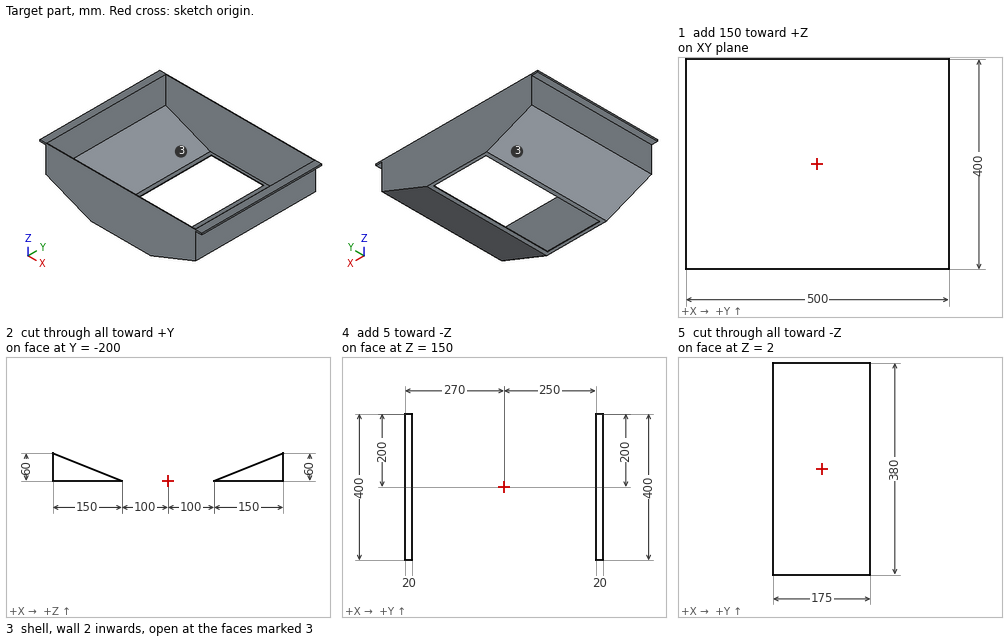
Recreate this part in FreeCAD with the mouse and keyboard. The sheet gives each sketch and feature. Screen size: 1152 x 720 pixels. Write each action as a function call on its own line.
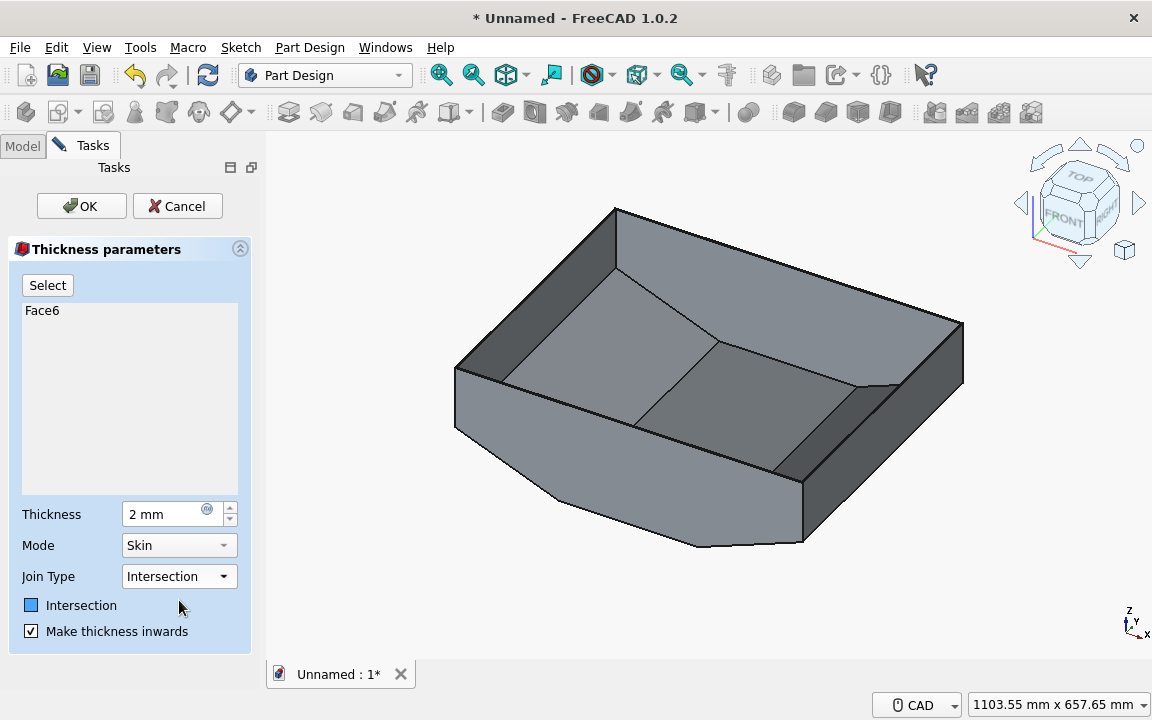
click(82, 206)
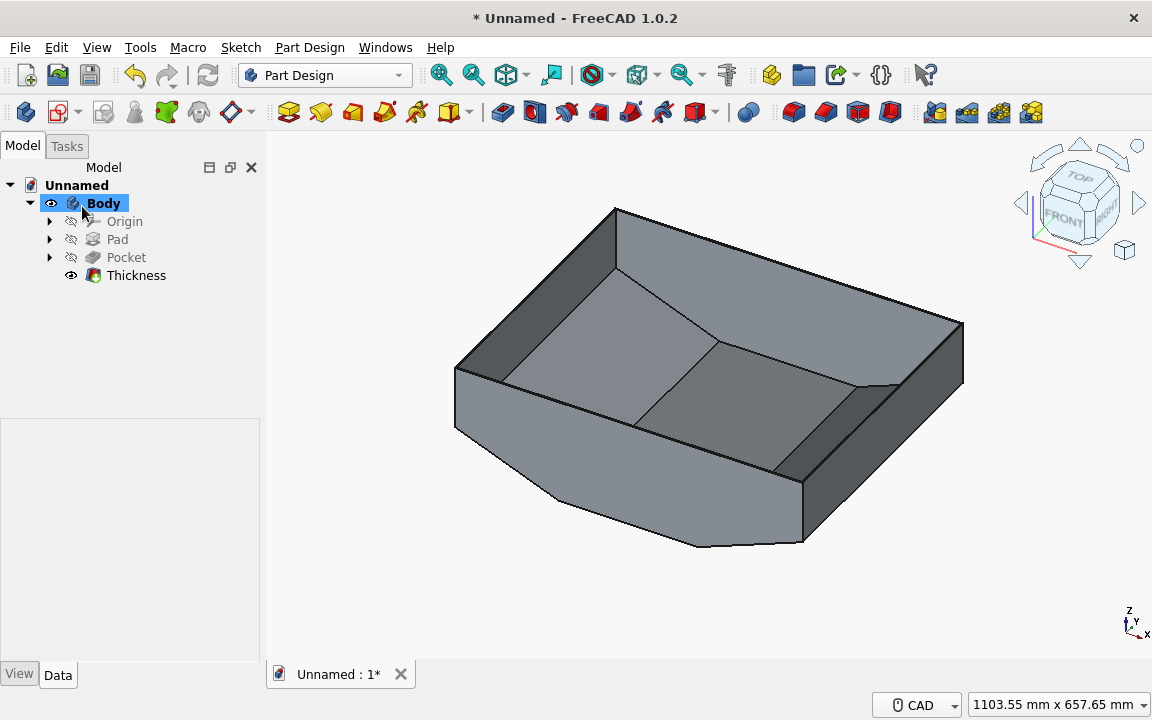
scroll(856, 428, up, 15)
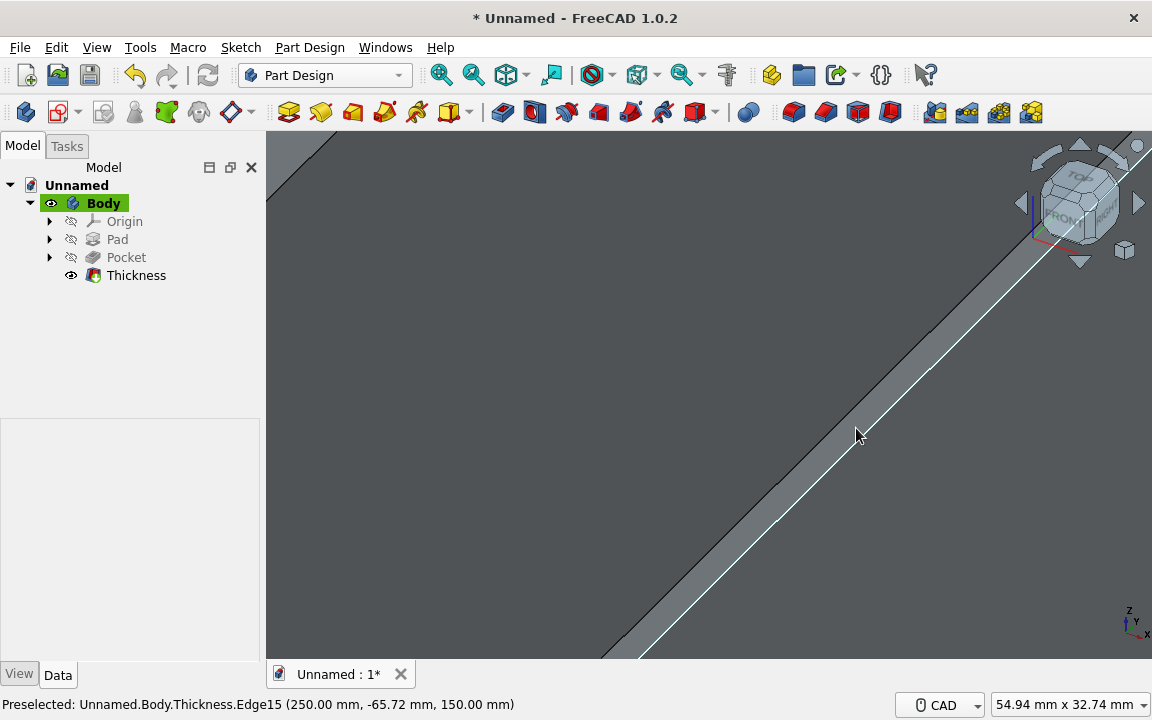
key(v)
key(f)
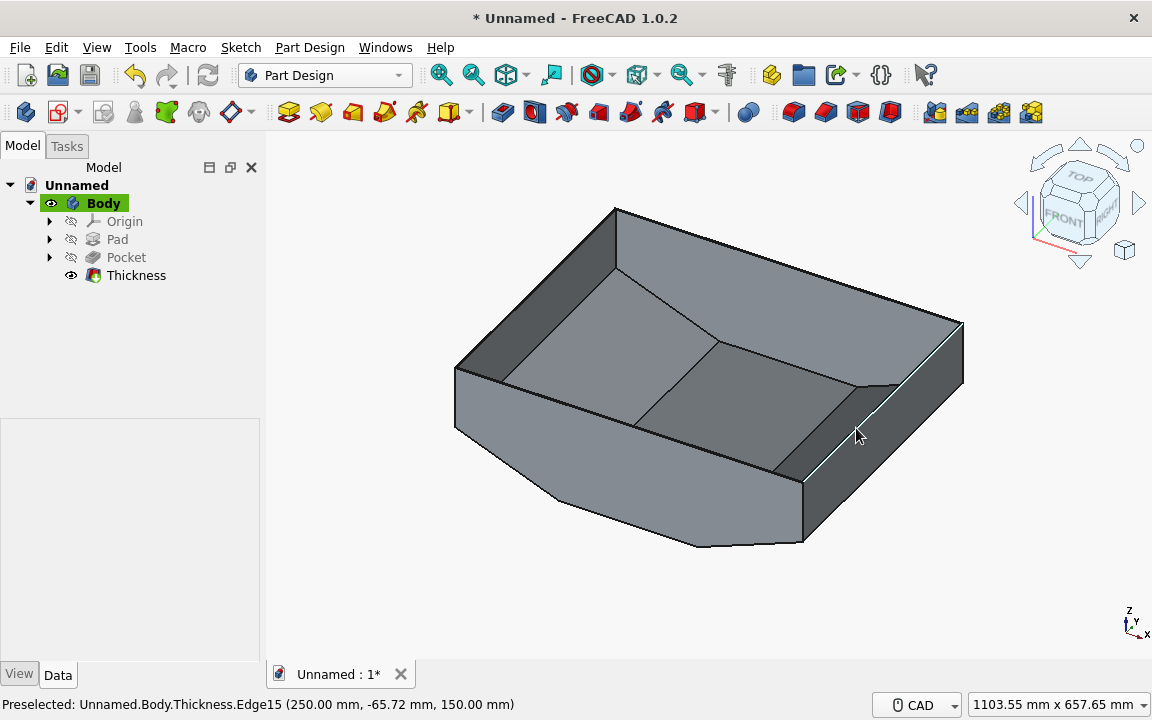
key(0)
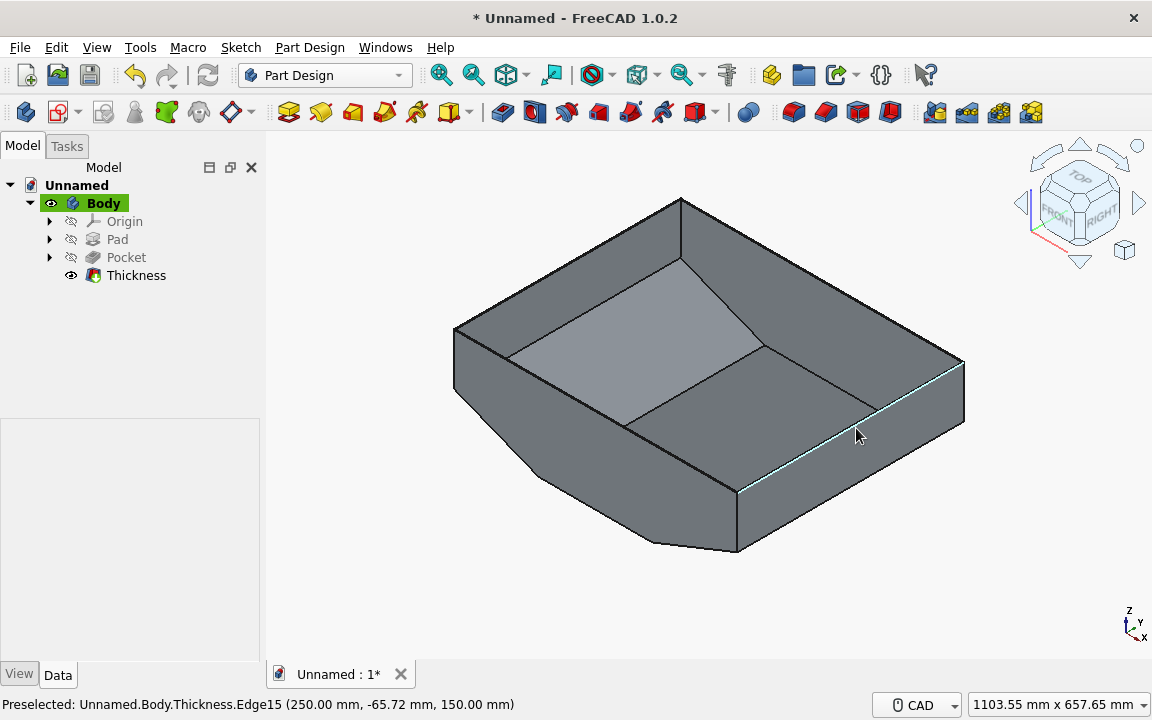
scroll(813, 448, up, 15)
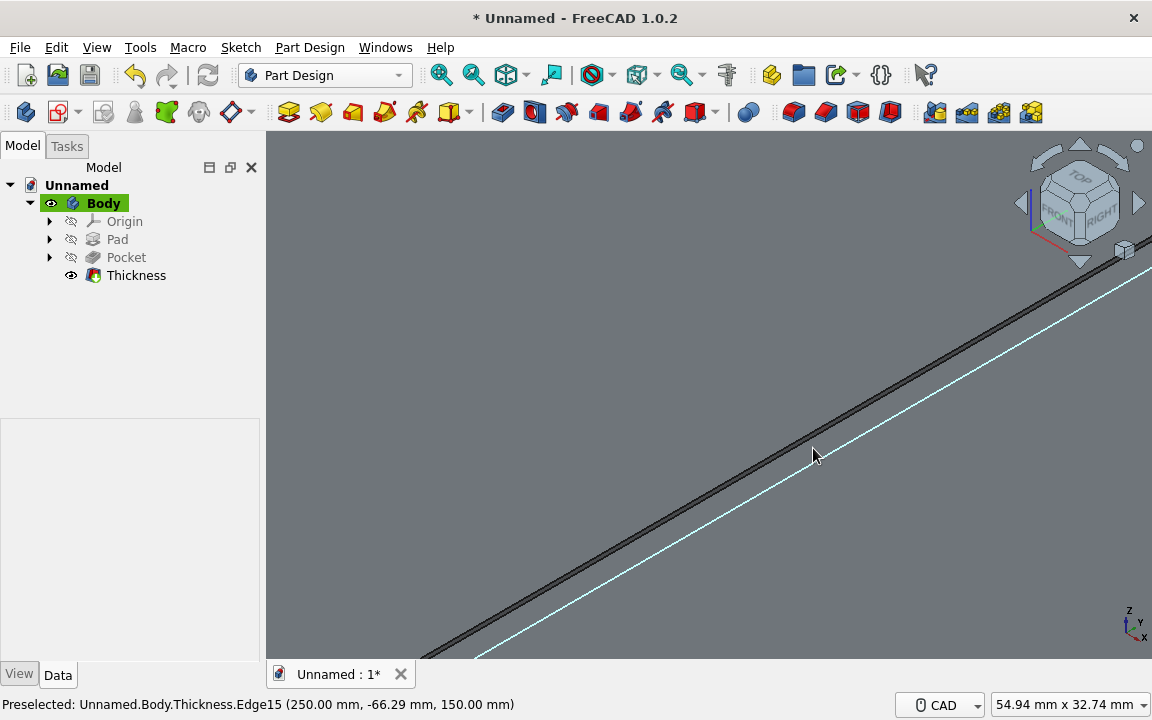
key(v)
key(f)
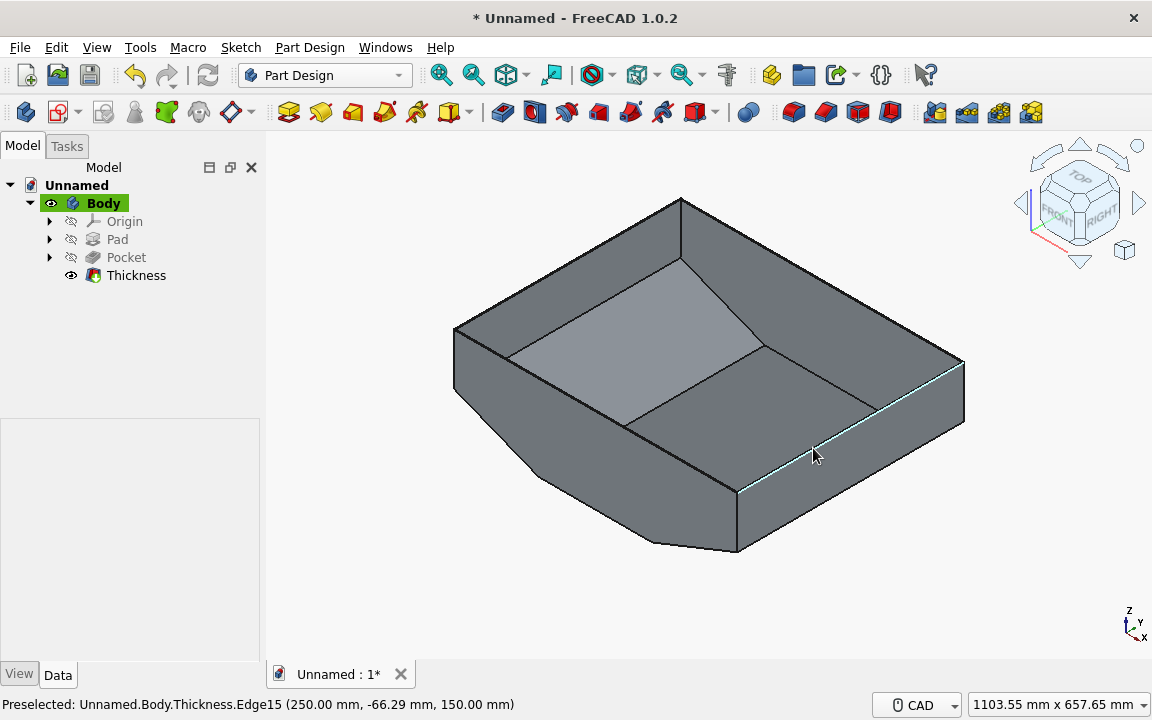
key(2)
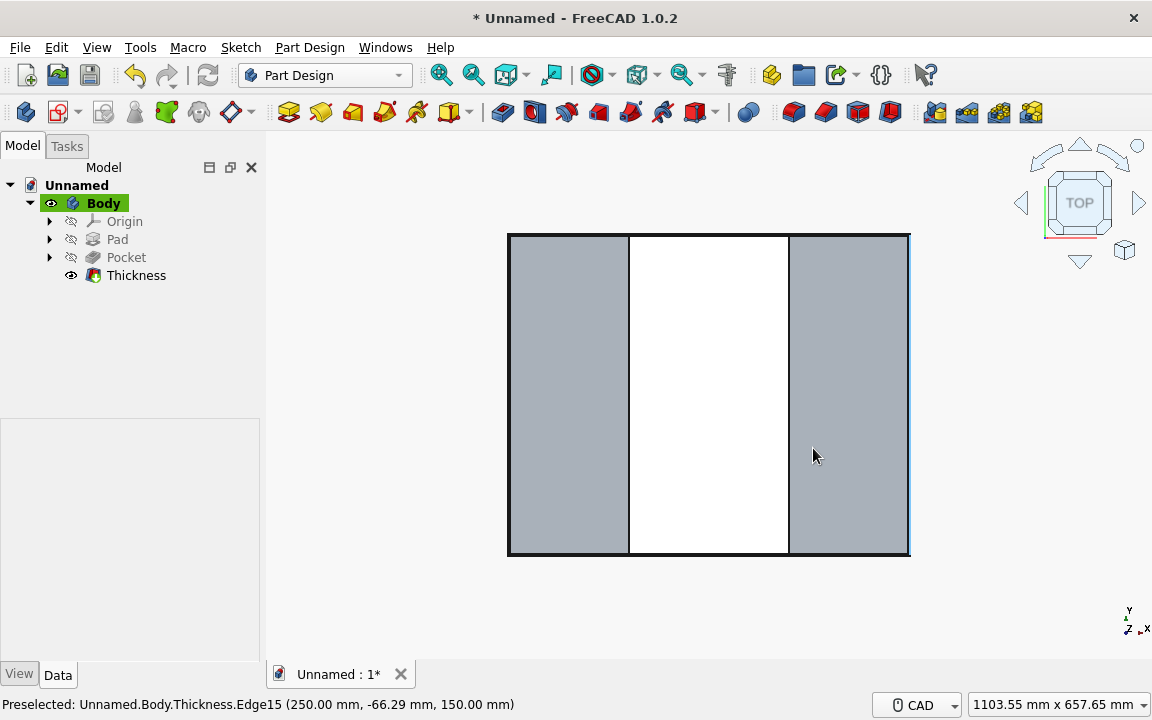
scroll(909, 447, up, 15)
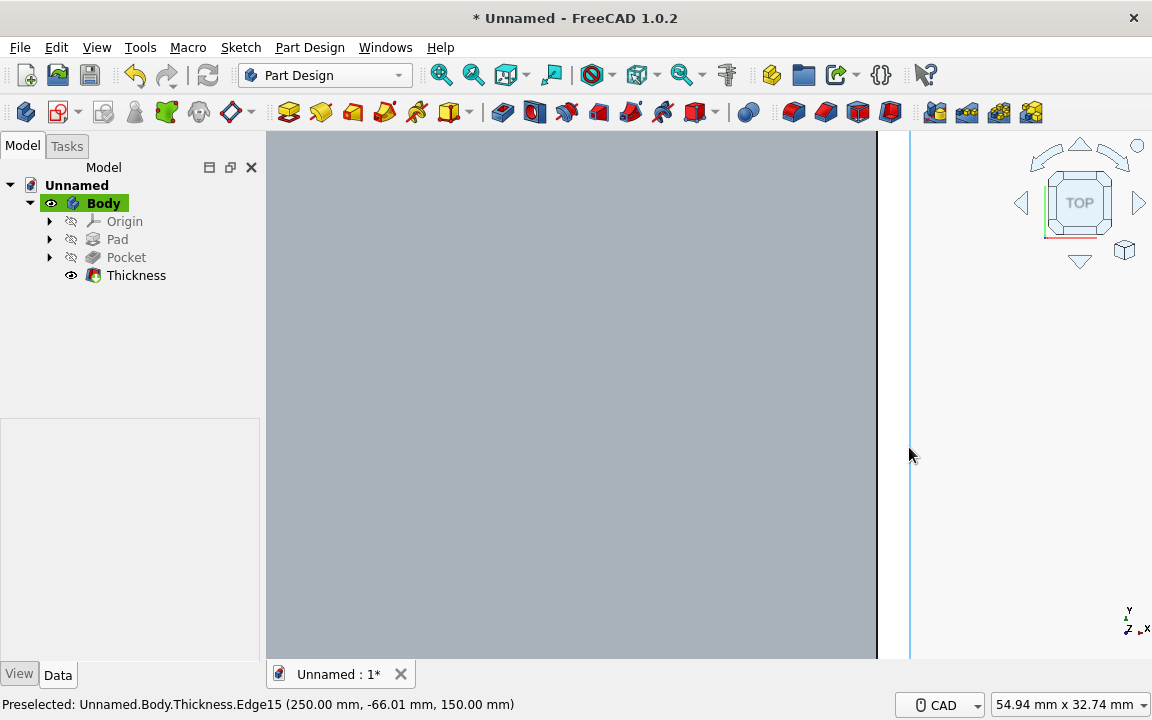
click(899, 454)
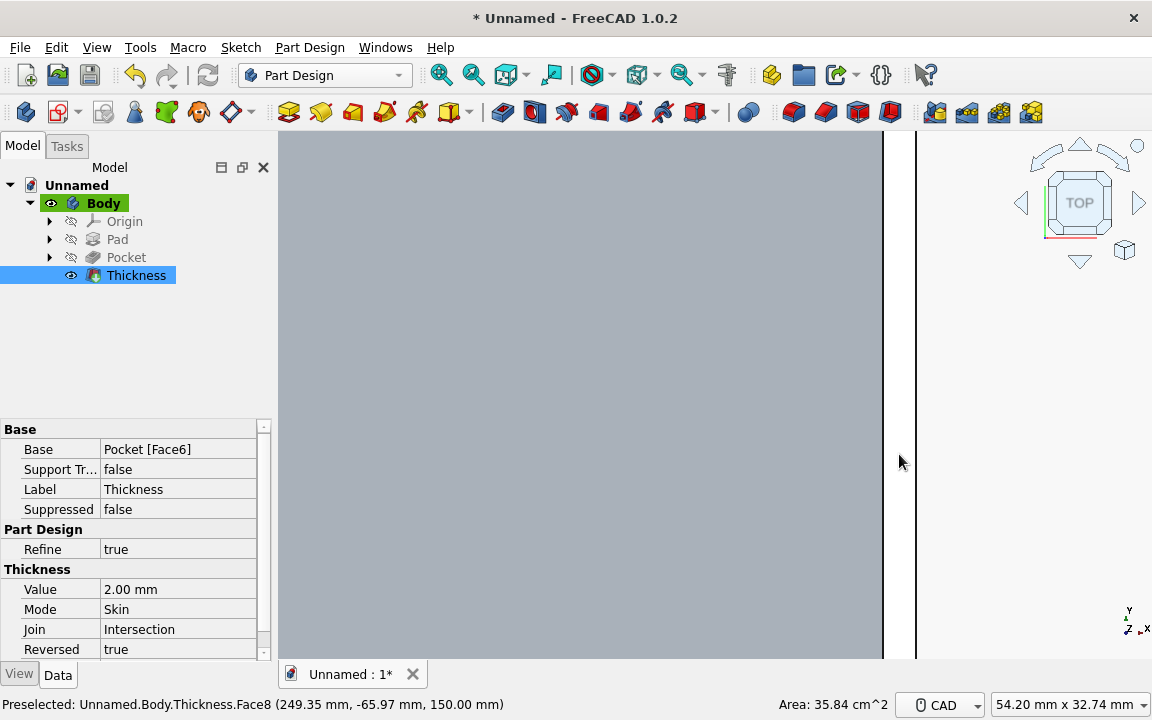
click(58, 112)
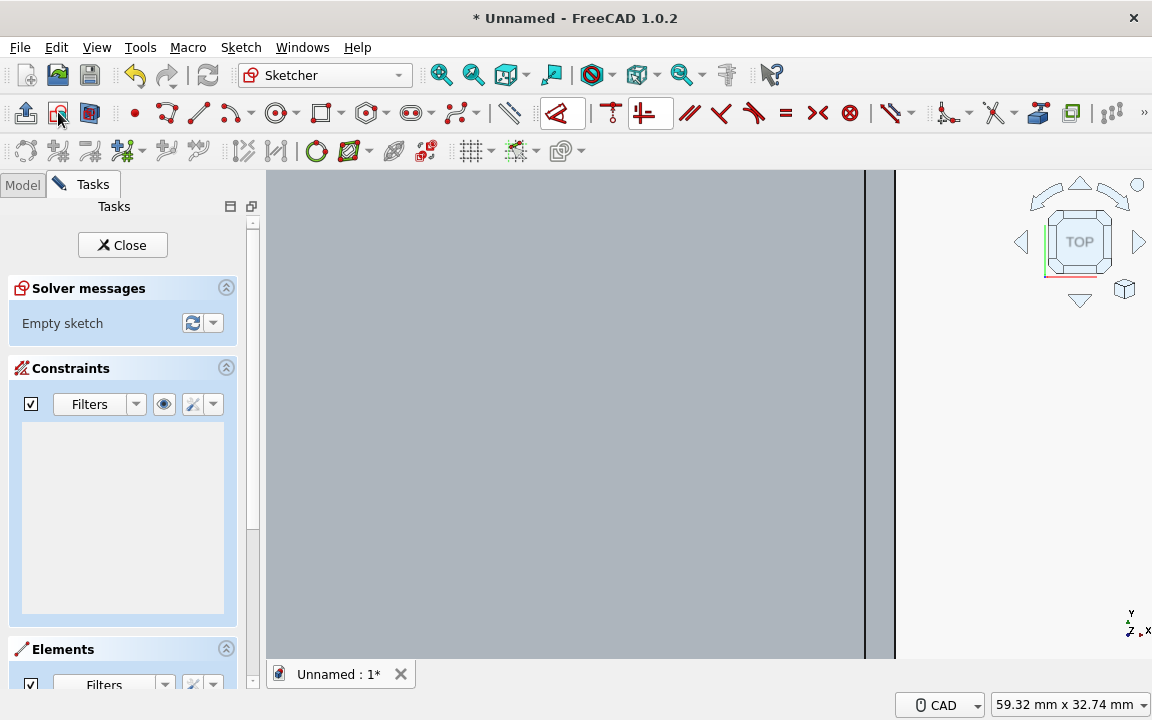
scroll(823, 463, down, 15)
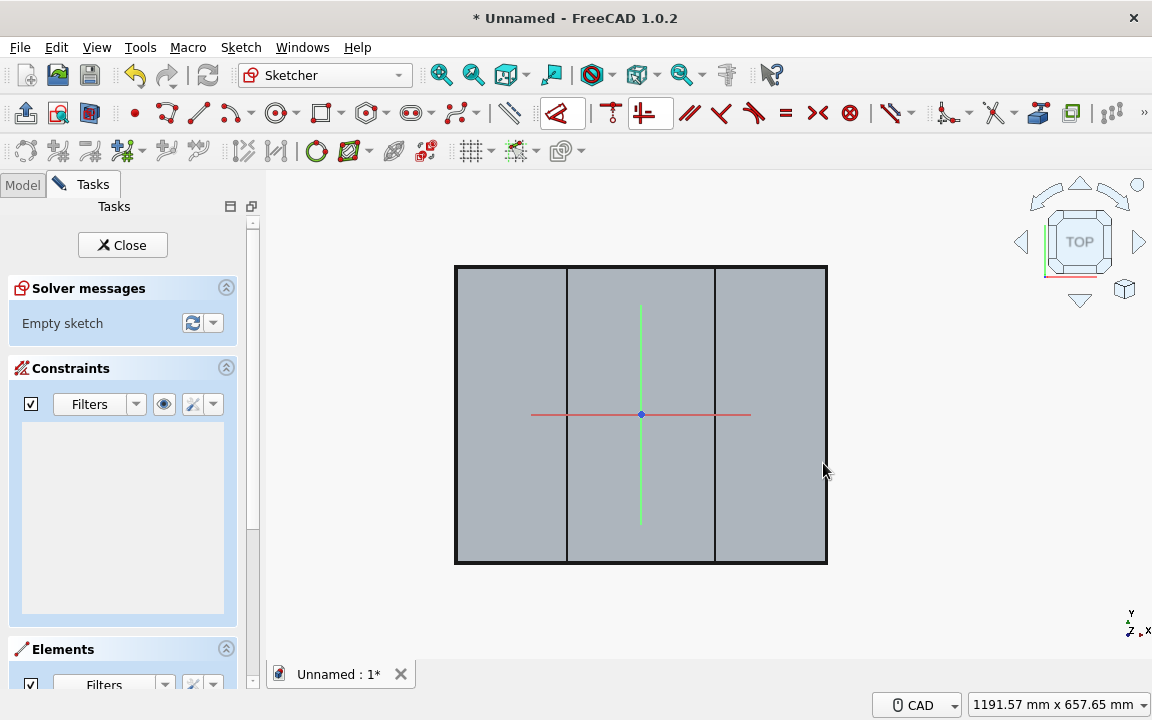
key(g)
key(r)